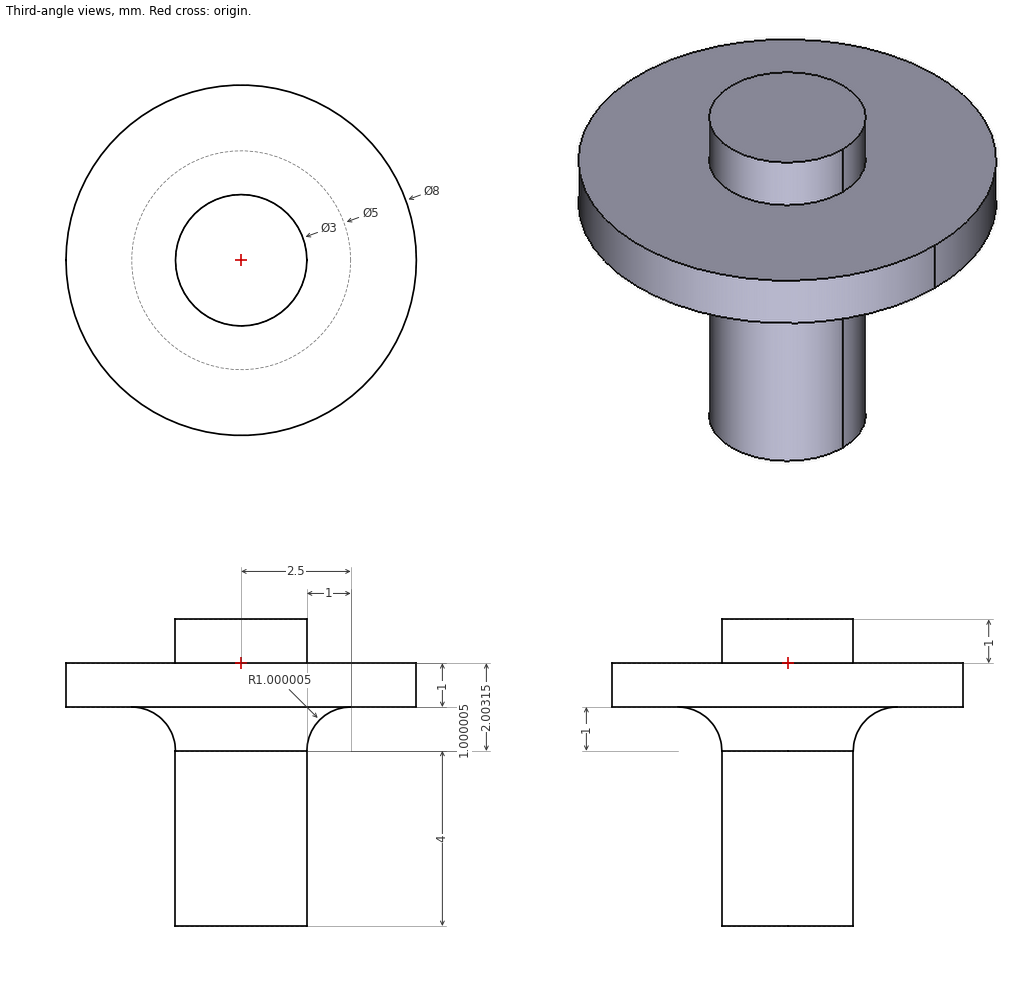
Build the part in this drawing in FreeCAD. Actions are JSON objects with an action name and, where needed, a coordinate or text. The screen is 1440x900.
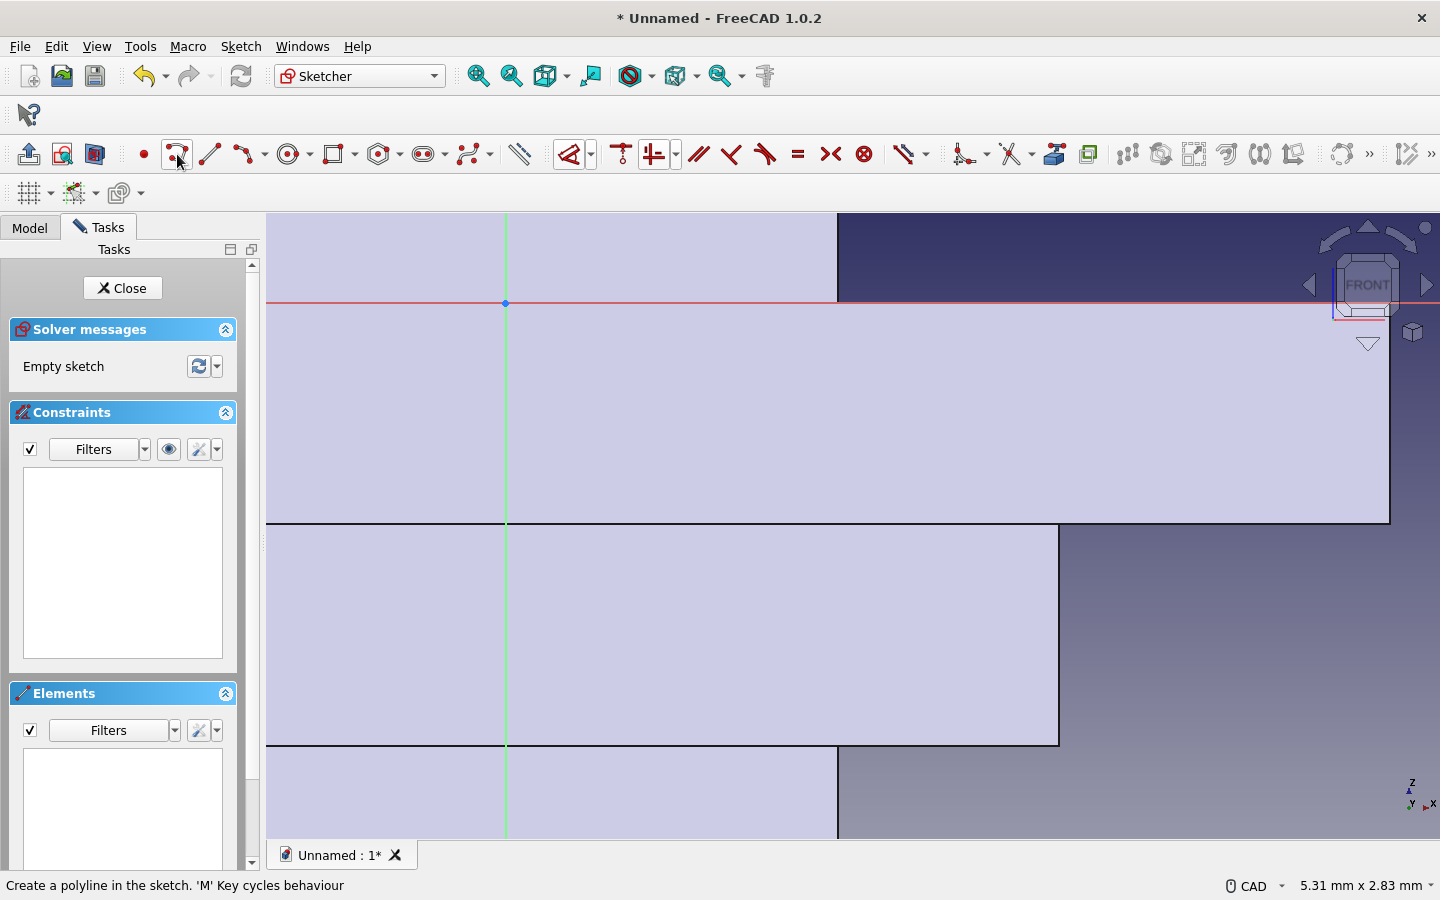
{"action": "left_click", "coordinate": [1059, 524]}
{"action": "left_click", "coordinate": [1059, 746]}
{"action": "left_click", "coordinate": [838, 757]}
{"action": "right_click", "coordinate": [838, 757]}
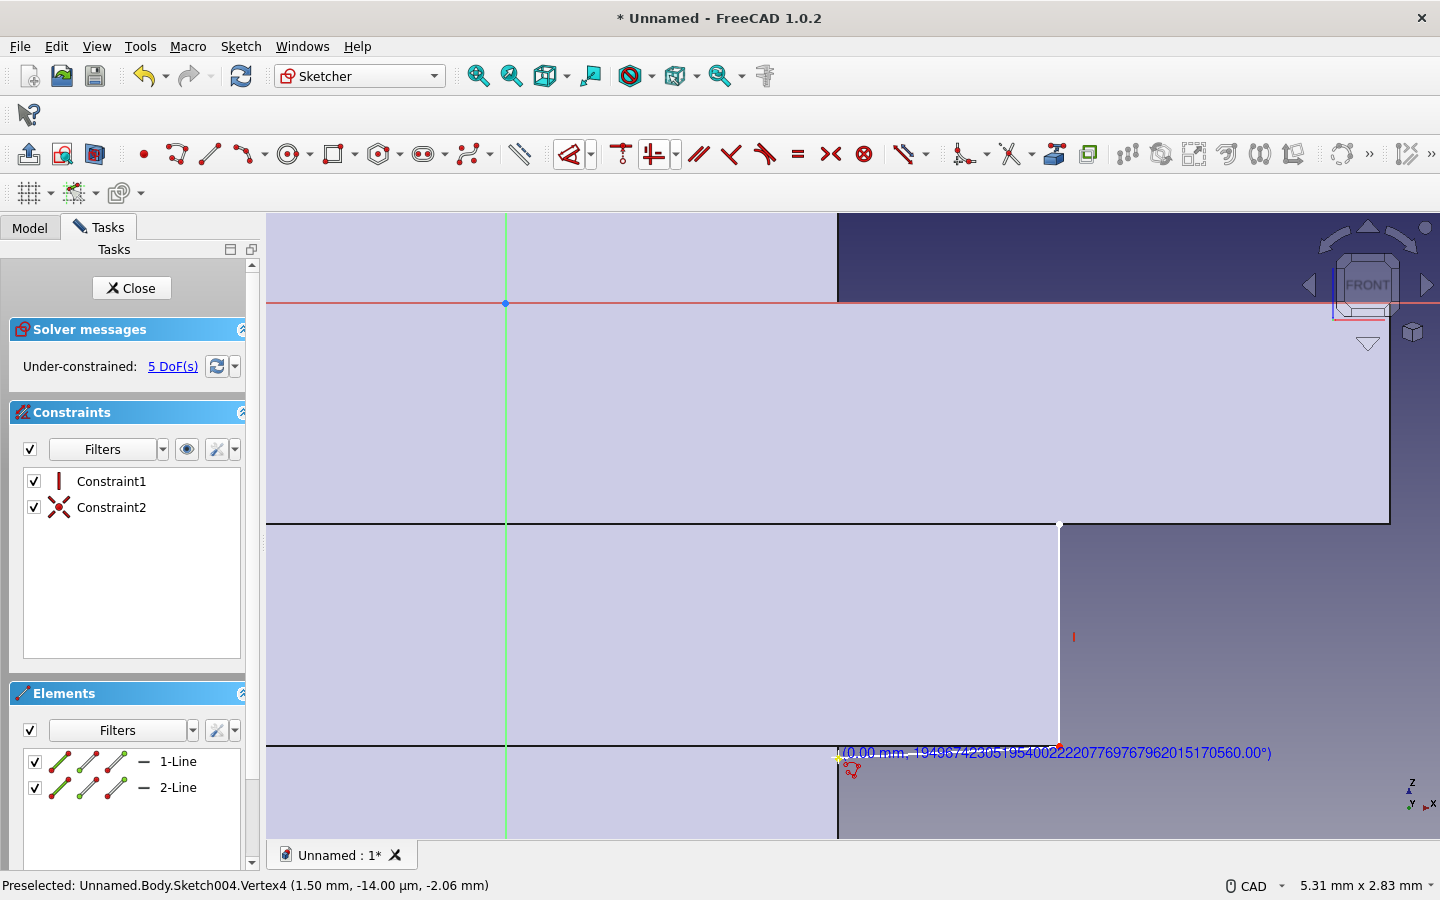
{"action": "left_click", "coordinate": [242, 154]}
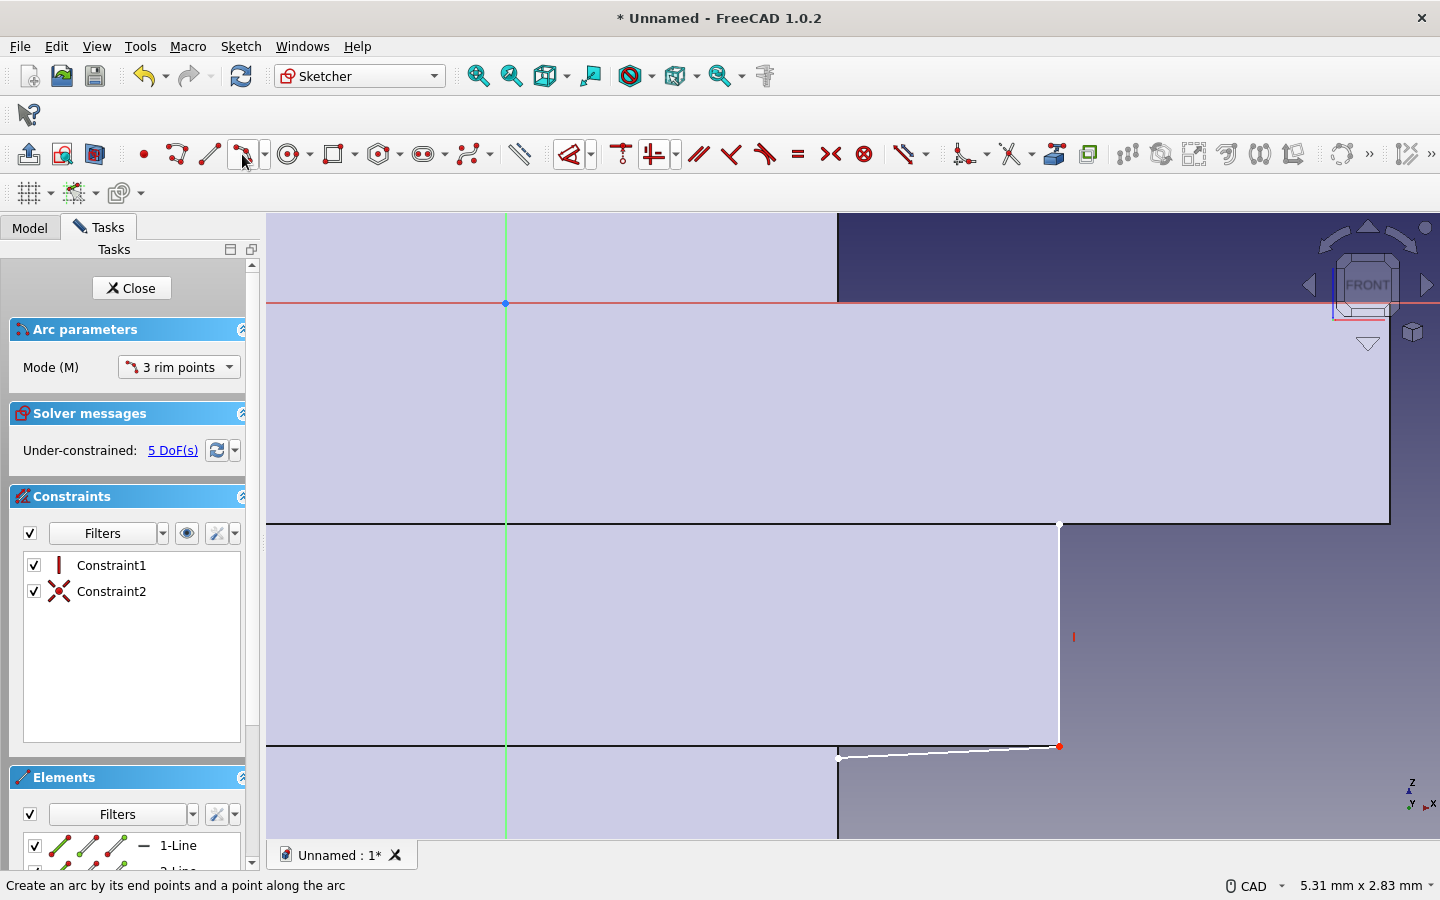
{"action": "left_click", "coordinate": [838, 758]}
{"action": "left_click", "coordinate": [1059, 525]}
{"action": "left_click", "coordinate": [902, 589]}
{"action": "key", "text": "Escape"}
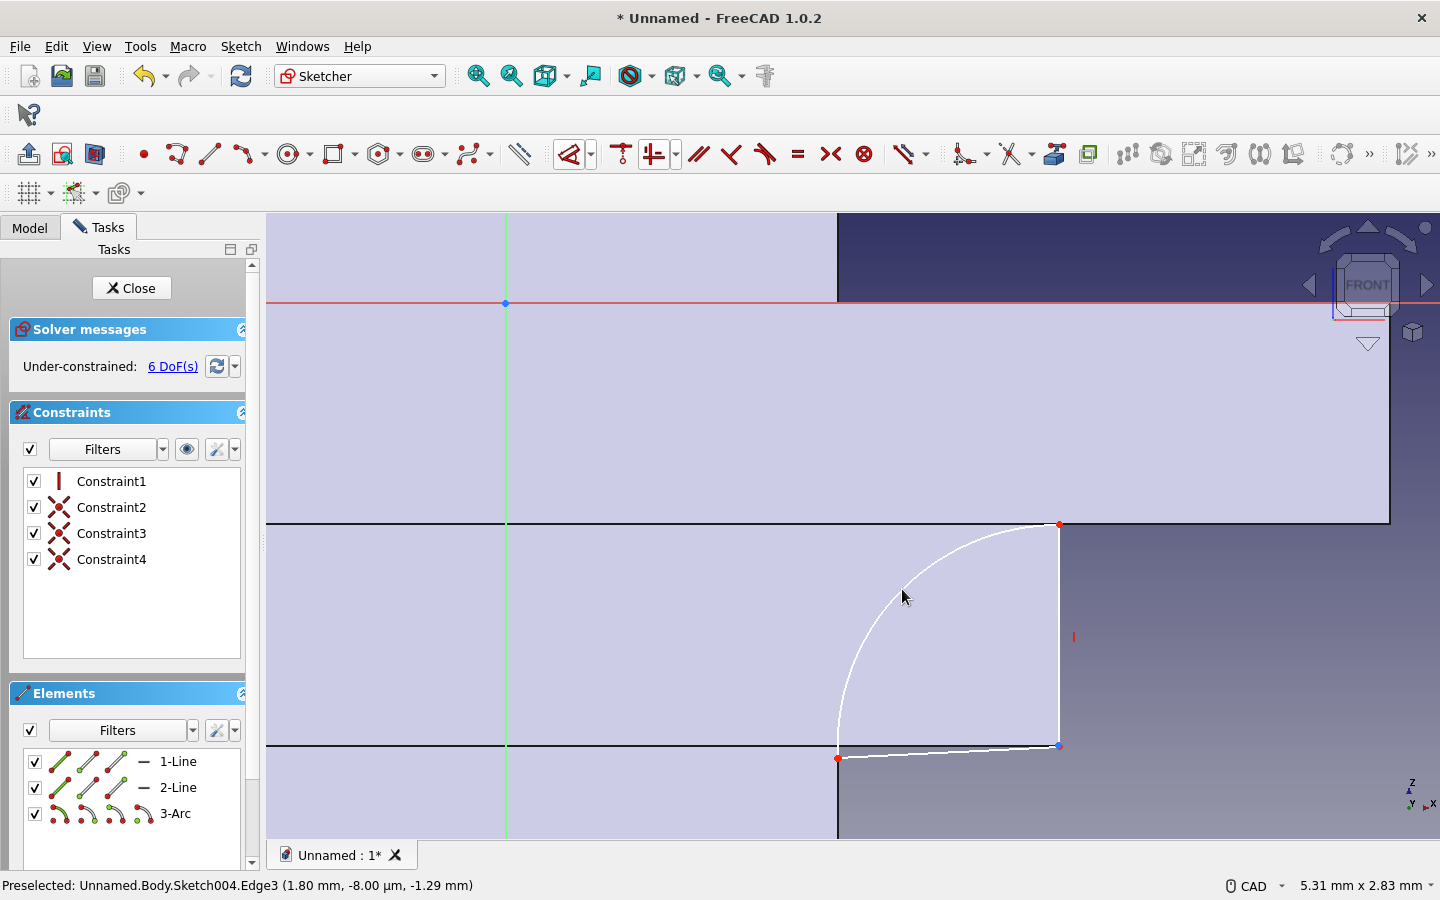
{"action": "left_click", "coordinate": [955, 551]}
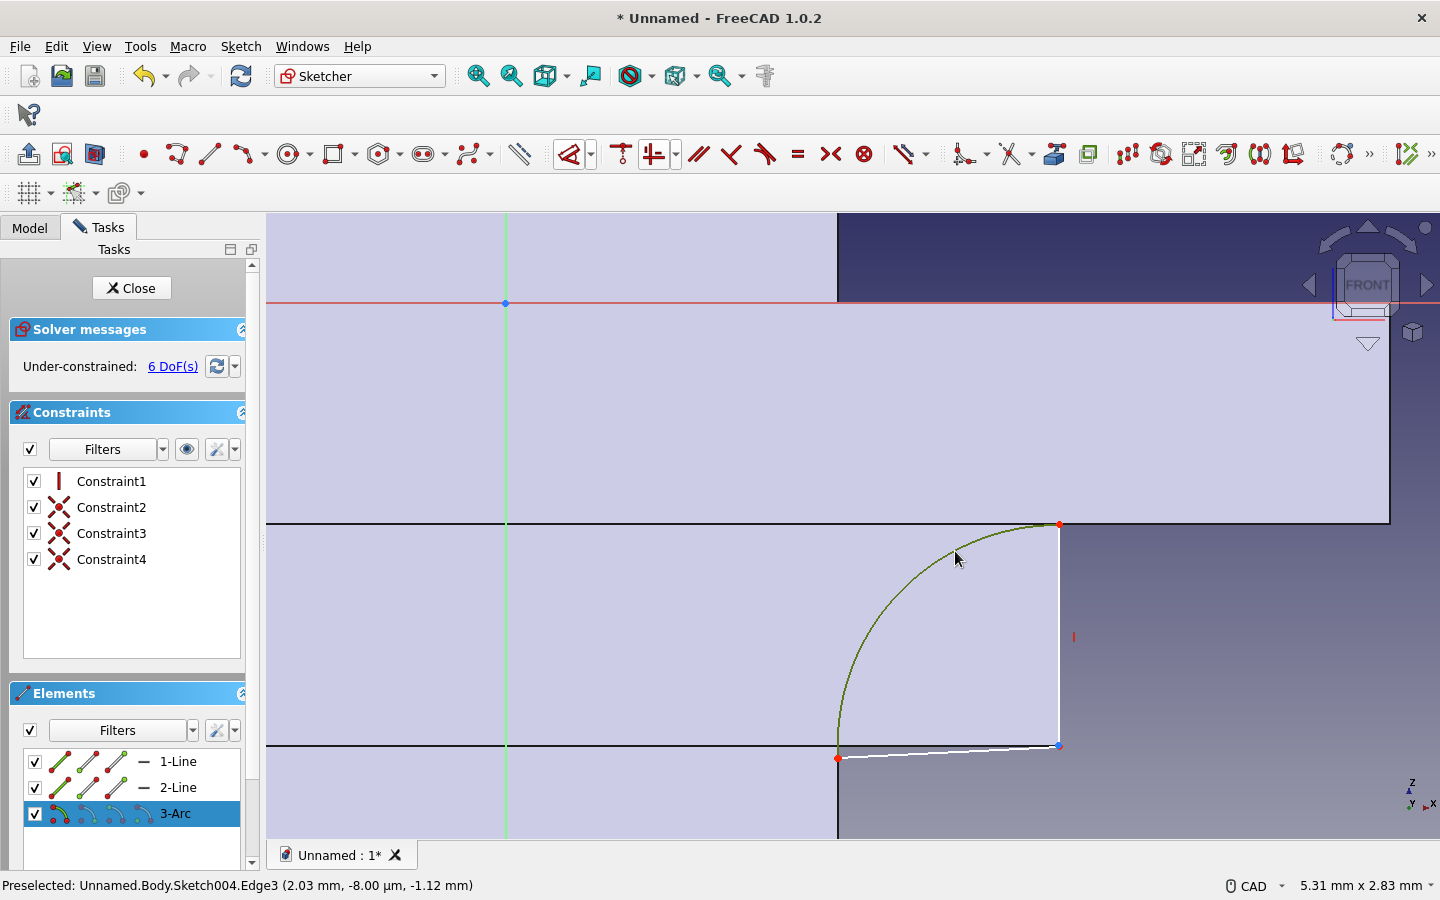
{"action": "key", "text": "k r"}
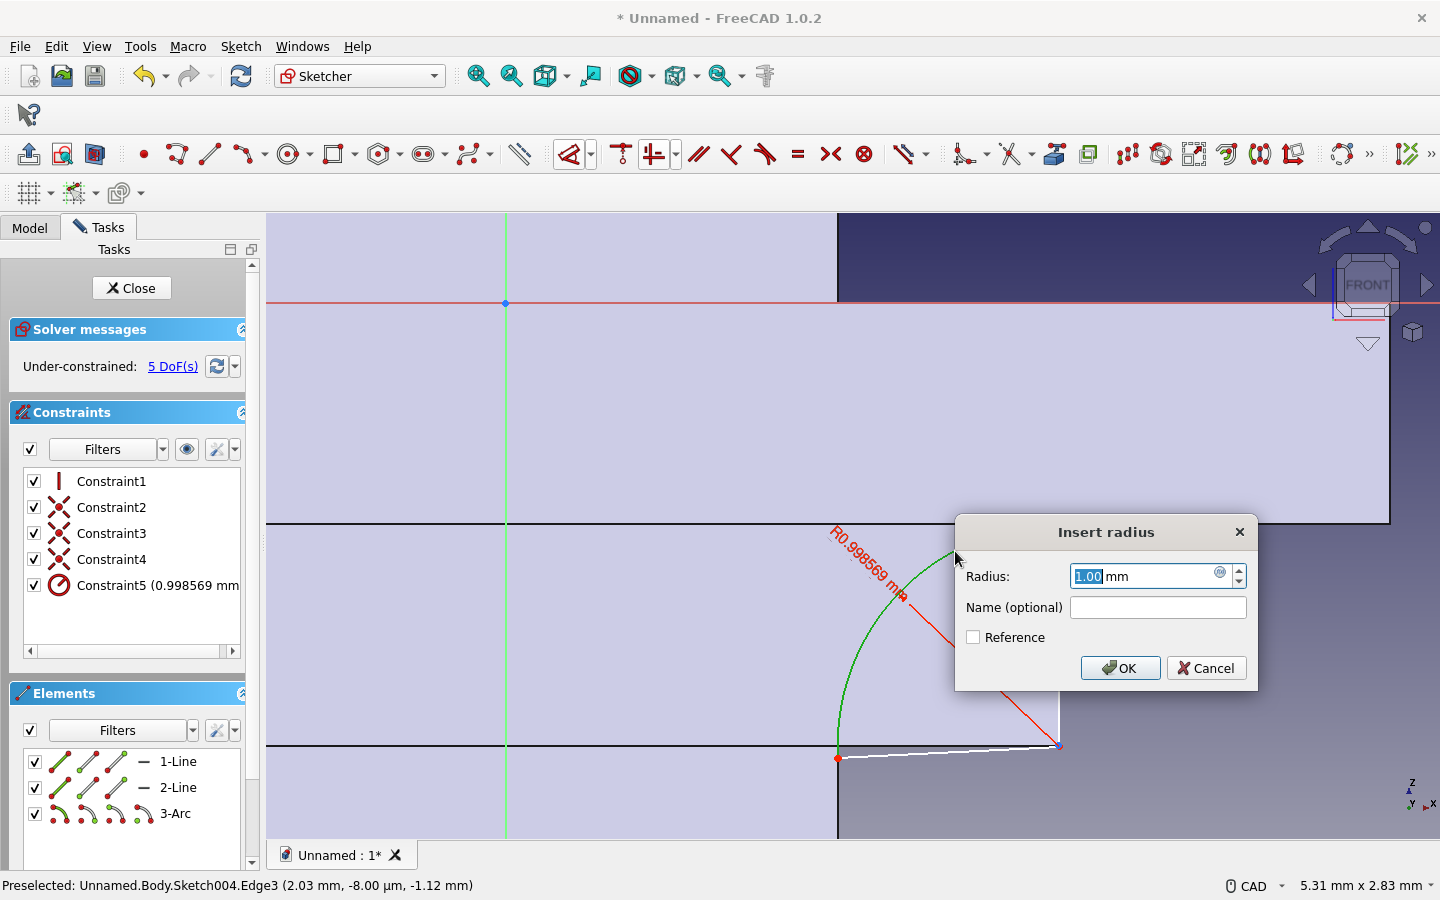
{"action": "type", "text": "1.000005"}
{"action": "key", "text": "Return"}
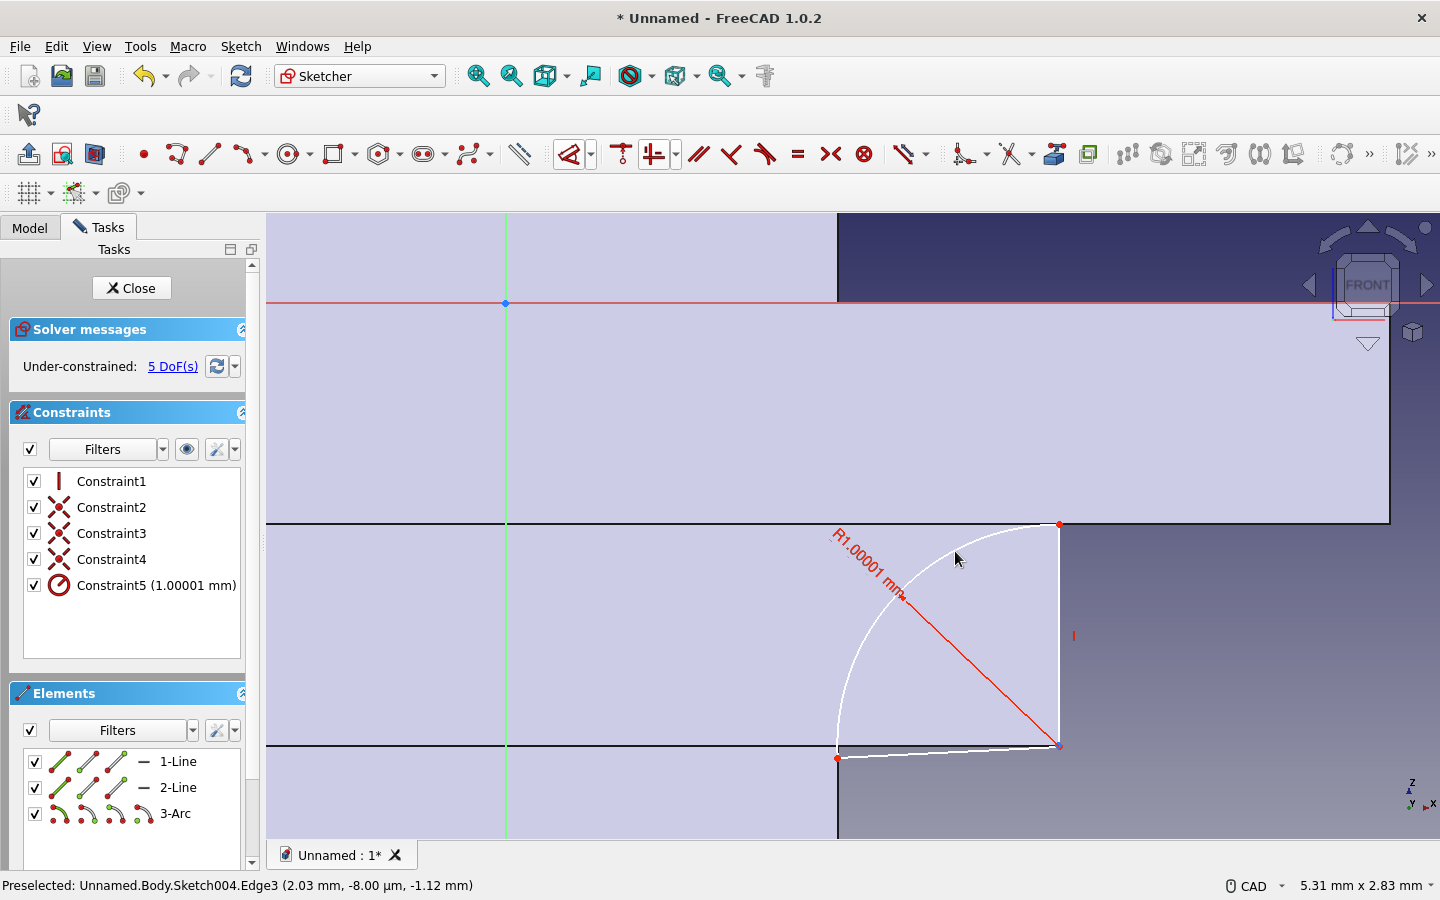
{"action": "left_click", "coordinate": [1059, 525]}